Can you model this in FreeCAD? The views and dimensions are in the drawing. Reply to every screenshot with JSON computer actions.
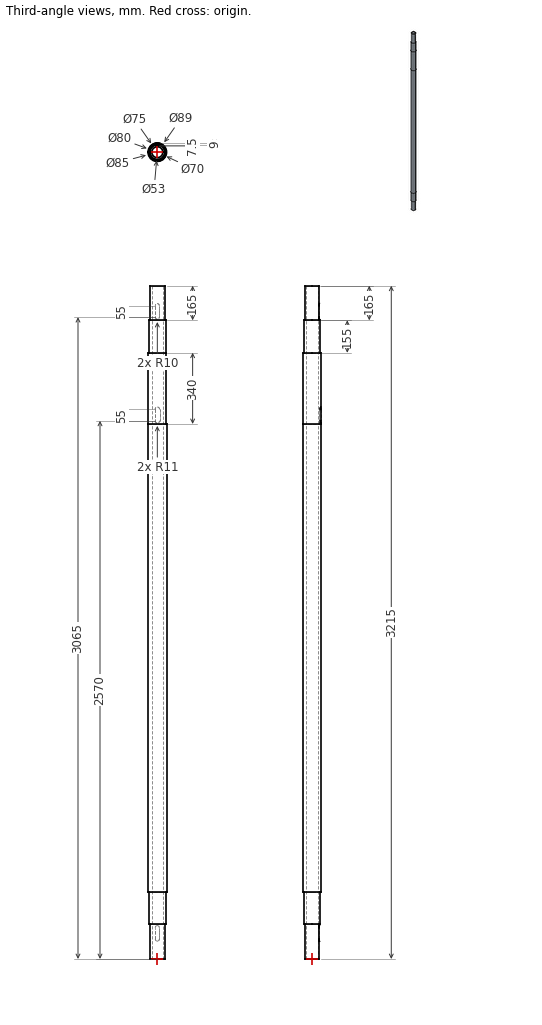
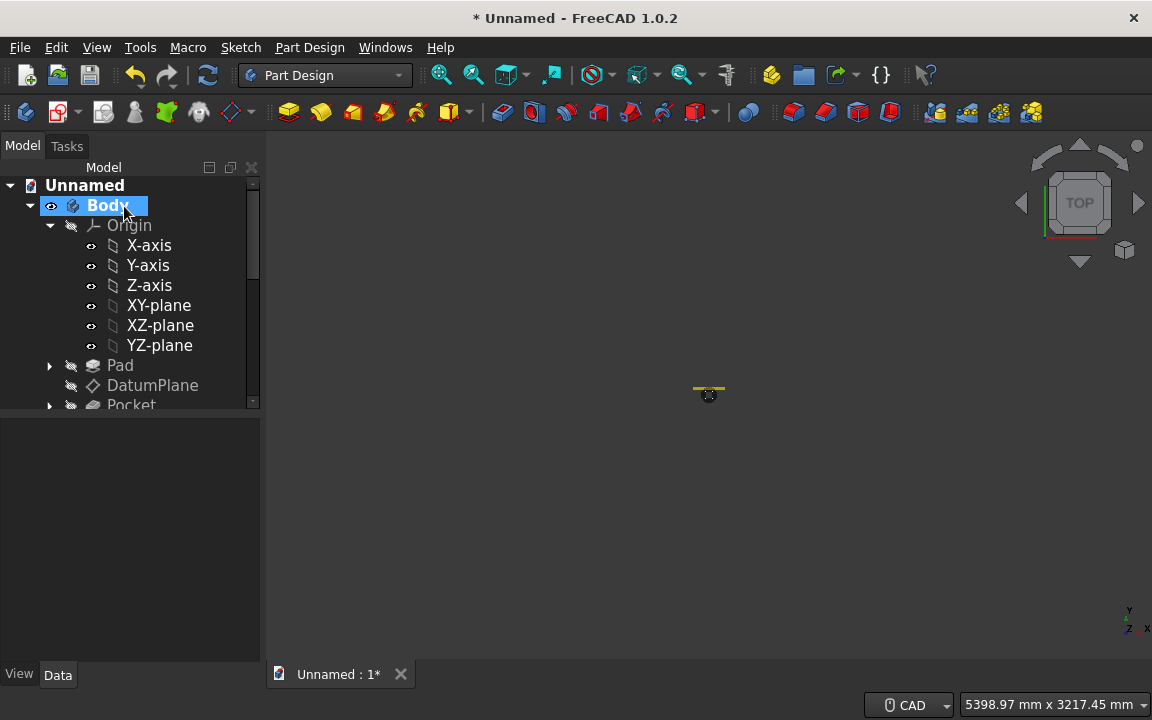
{"action": "scroll", "coordinate": [100, 301], "scroll_direction": "down", "scroll_amount": 3}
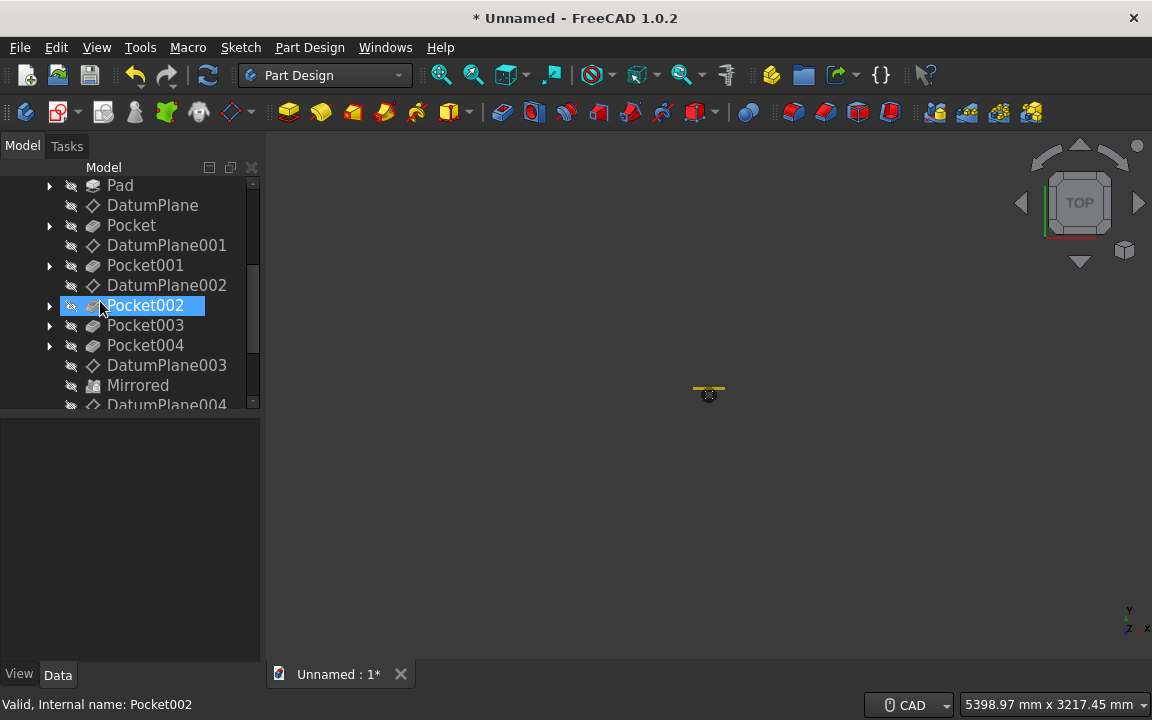
{"action": "scroll", "coordinate": [140, 301], "scroll_direction": "up", "scroll_amount": 15}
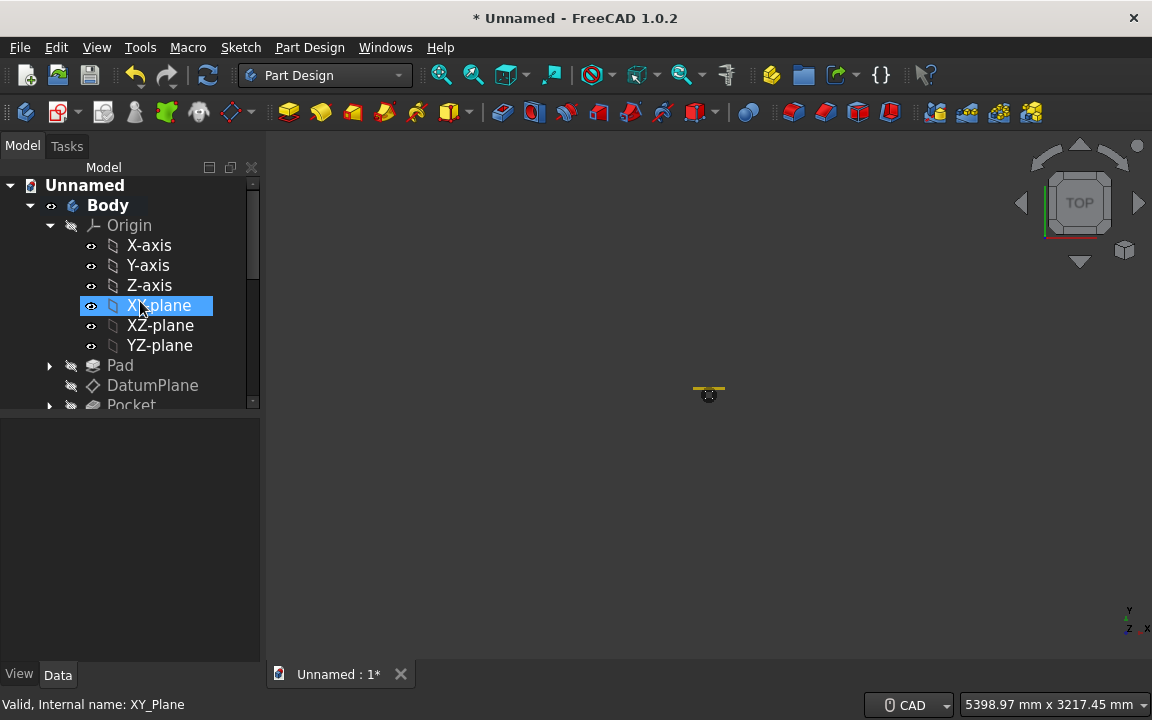
{"action": "scroll", "coordinate": [100, 301], "scroll_direction": "down", "scroll_amount": 6}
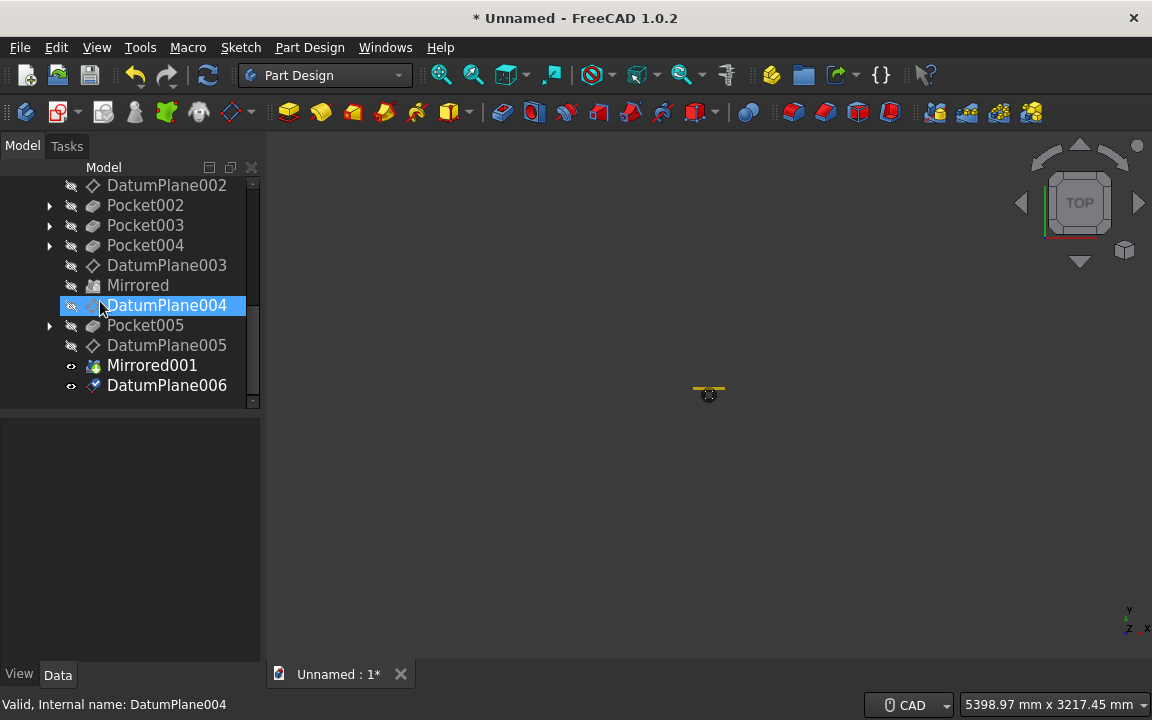
{"action": "left_click", "coordinate": [116, 386]}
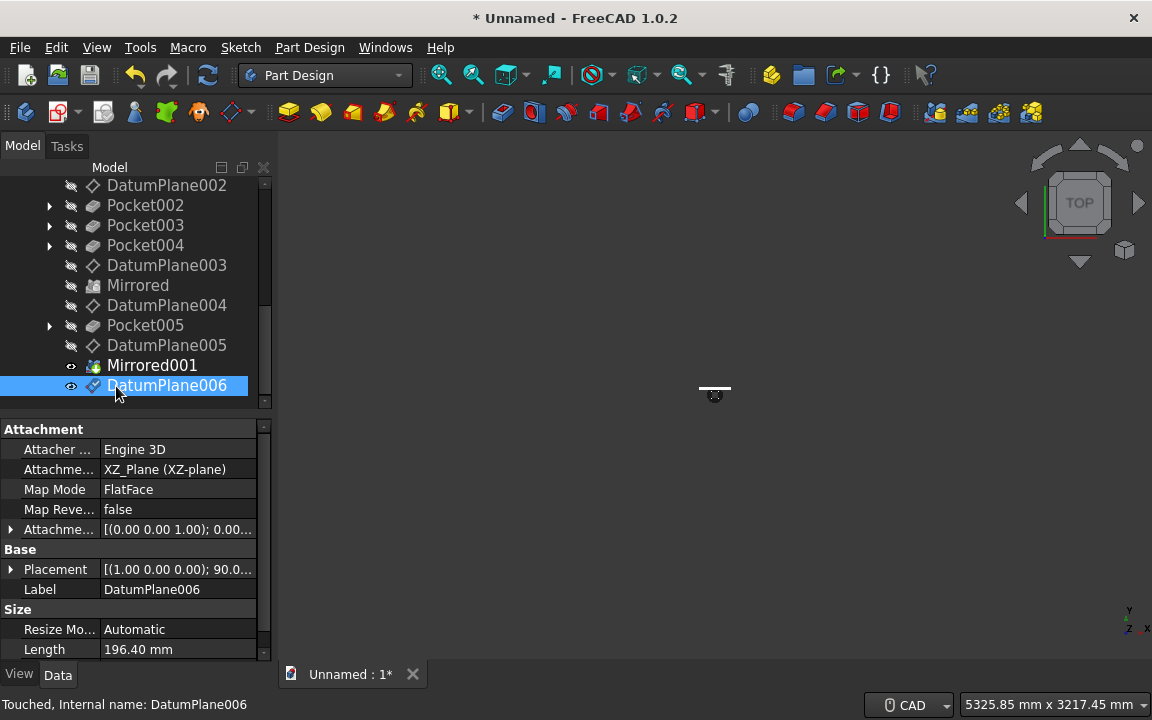
{"action": "left_click", "coordinate": [58, 112]}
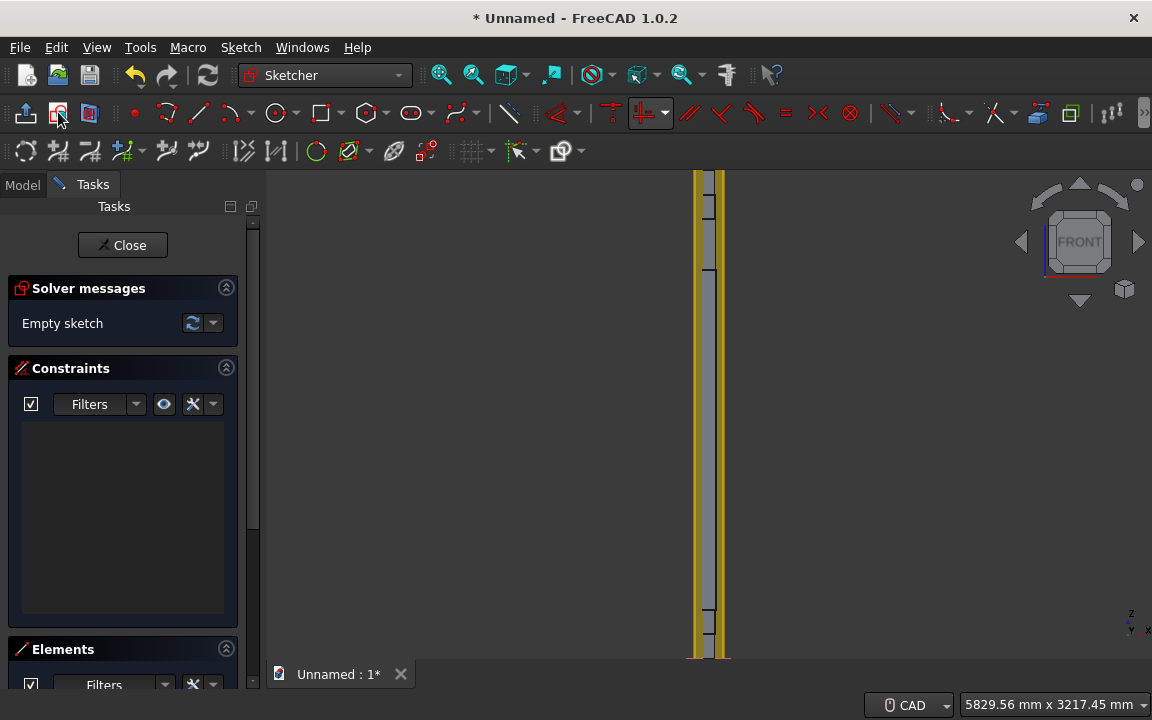
{"action": "left_click", "coordinate": [90, 114]}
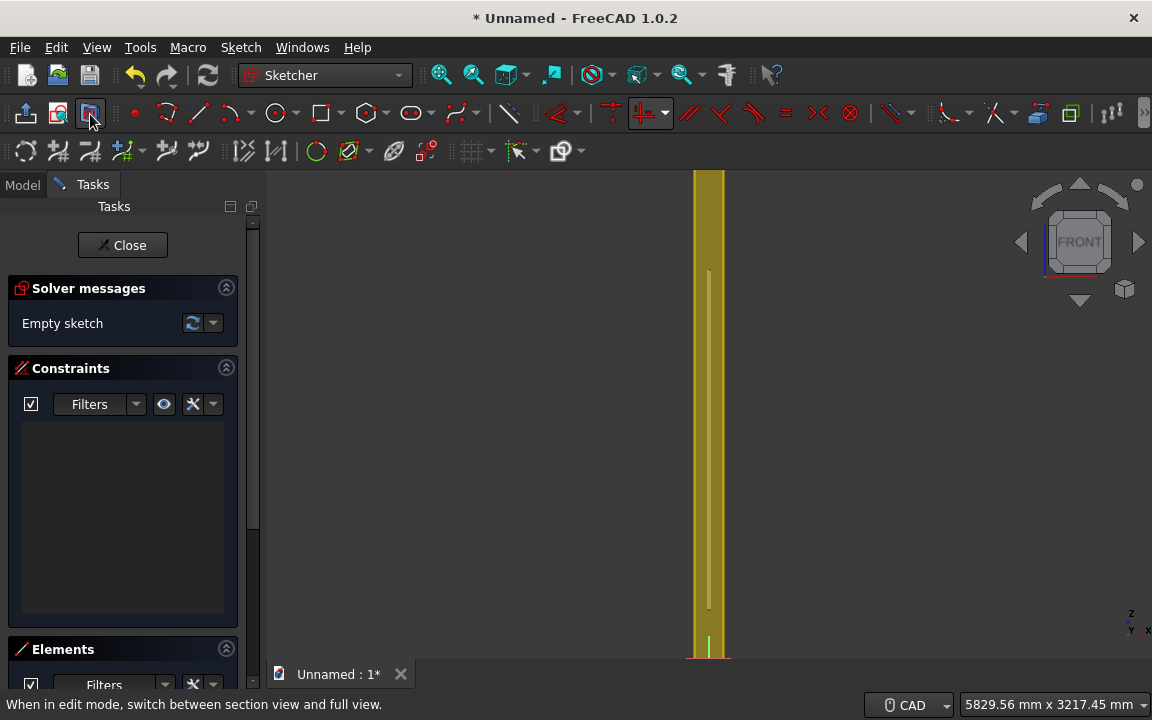
{"action": "scroll", "coordinate": [713, 256], "scroll_direction": "up", "scroll_amount": 15}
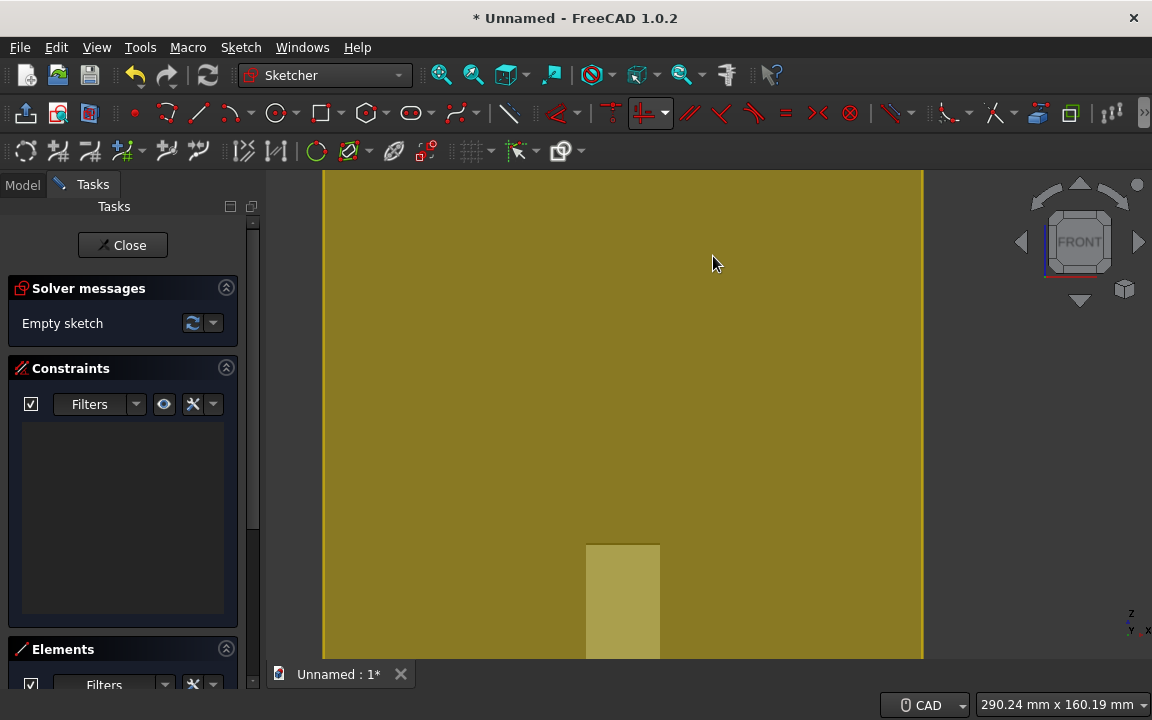
{"action": "left_click", "coordinate": [412, 114]}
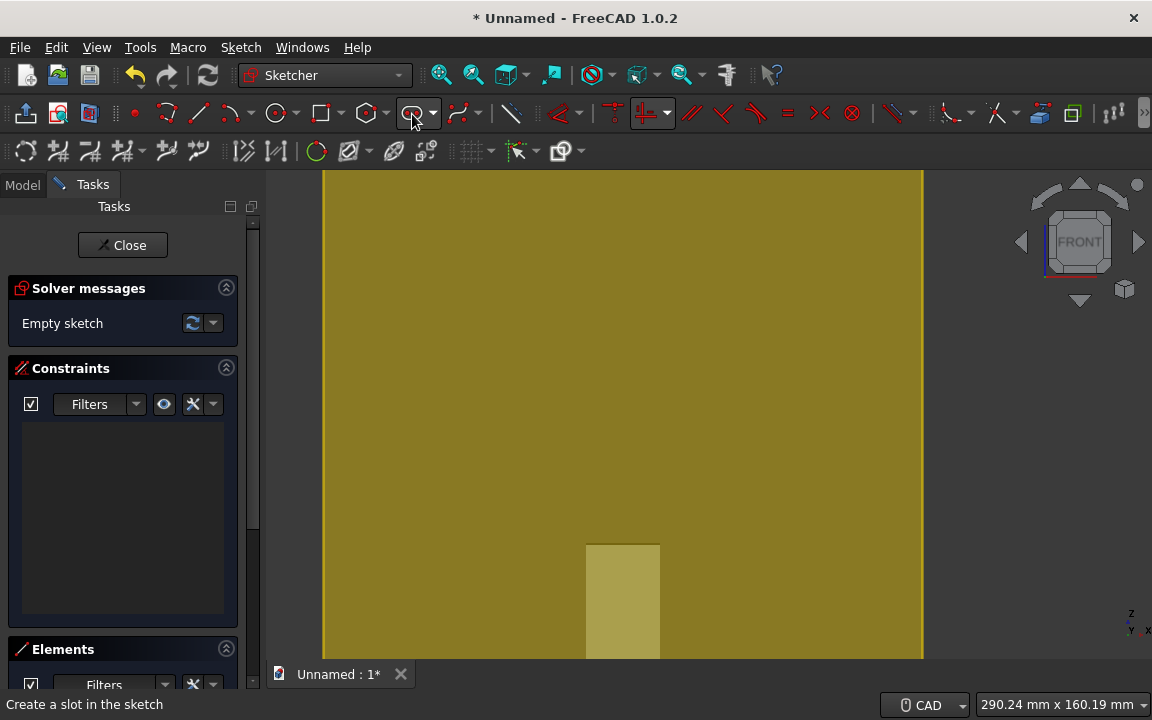
{"action": "left_click", "coordinate": [623, 498]}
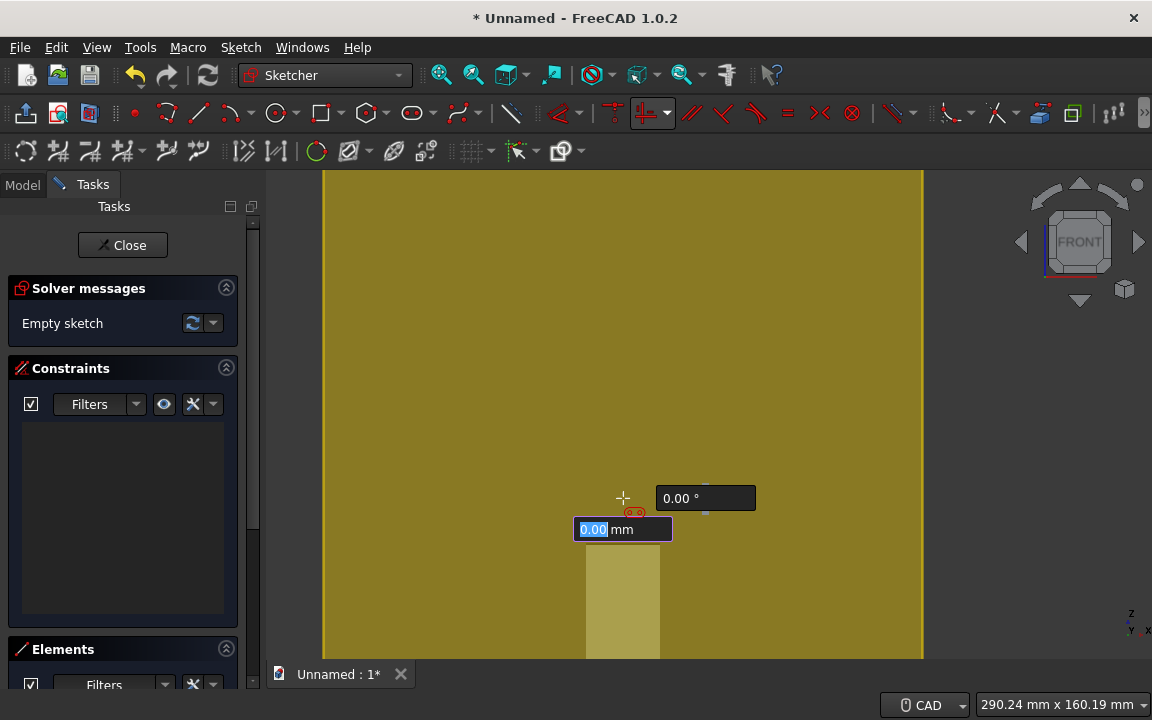
{"action": "left_click", "coordinate": [632, 330]}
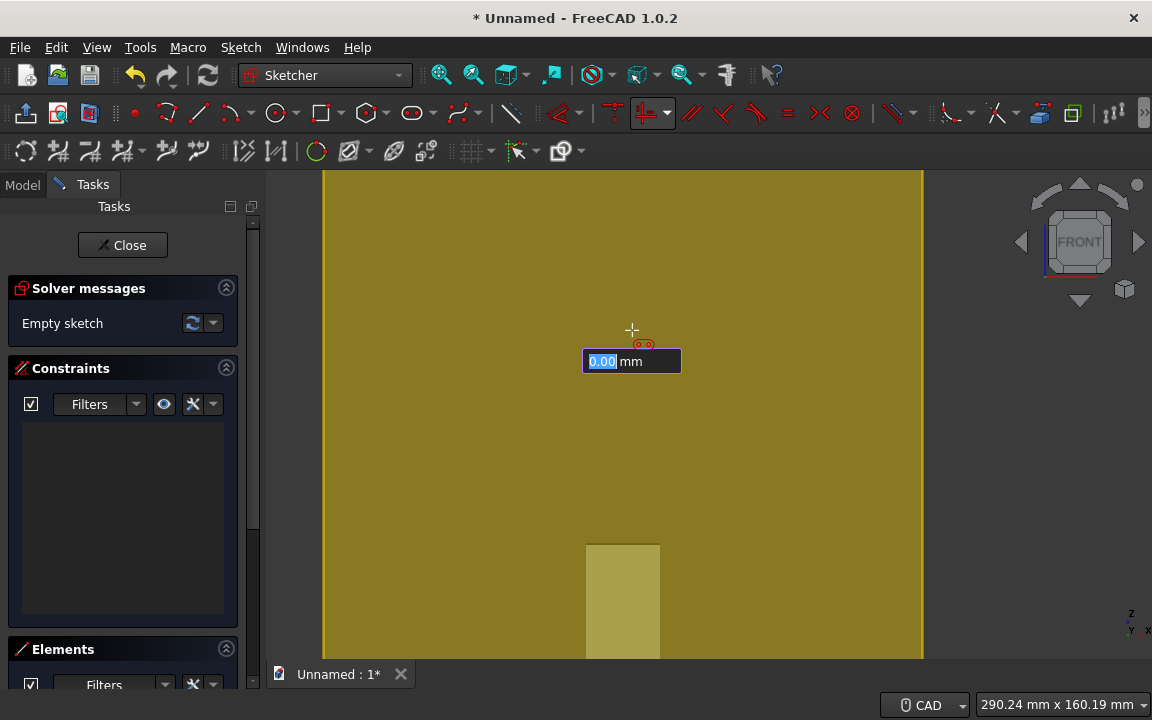
{"action": "left_click", "coordinate": [657, 414]}
{"action": "key", "text": "Escape"}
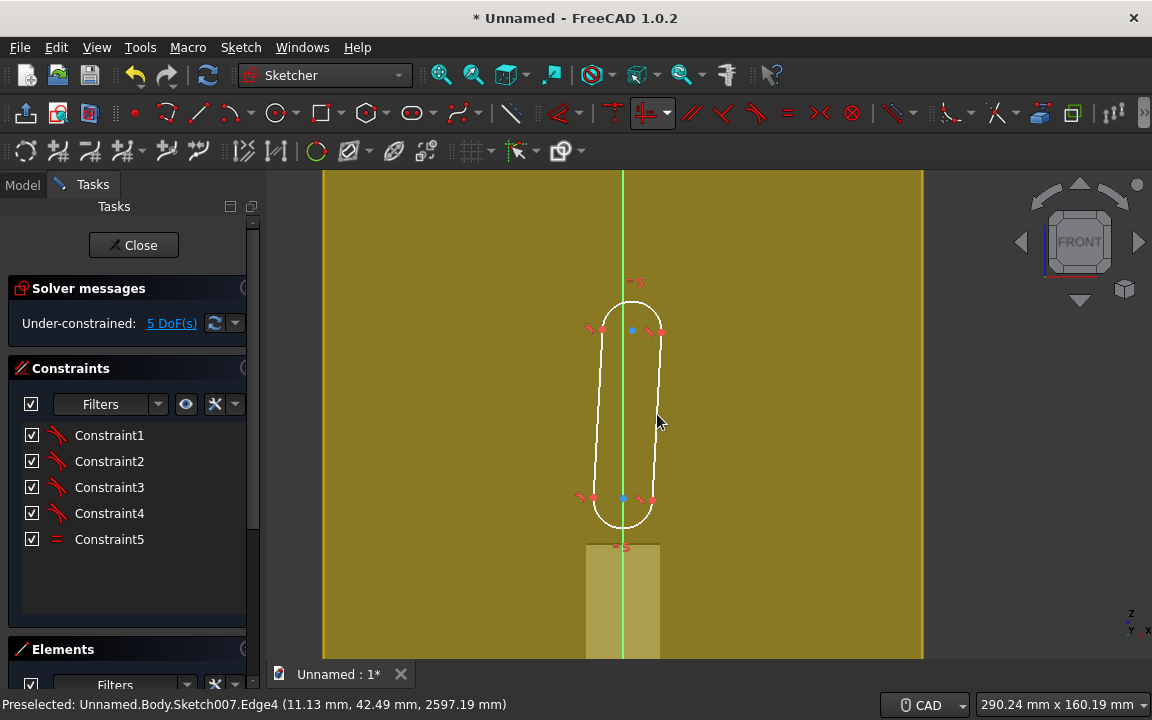
{"action": "left_click", "coordinate": [596, 447]}